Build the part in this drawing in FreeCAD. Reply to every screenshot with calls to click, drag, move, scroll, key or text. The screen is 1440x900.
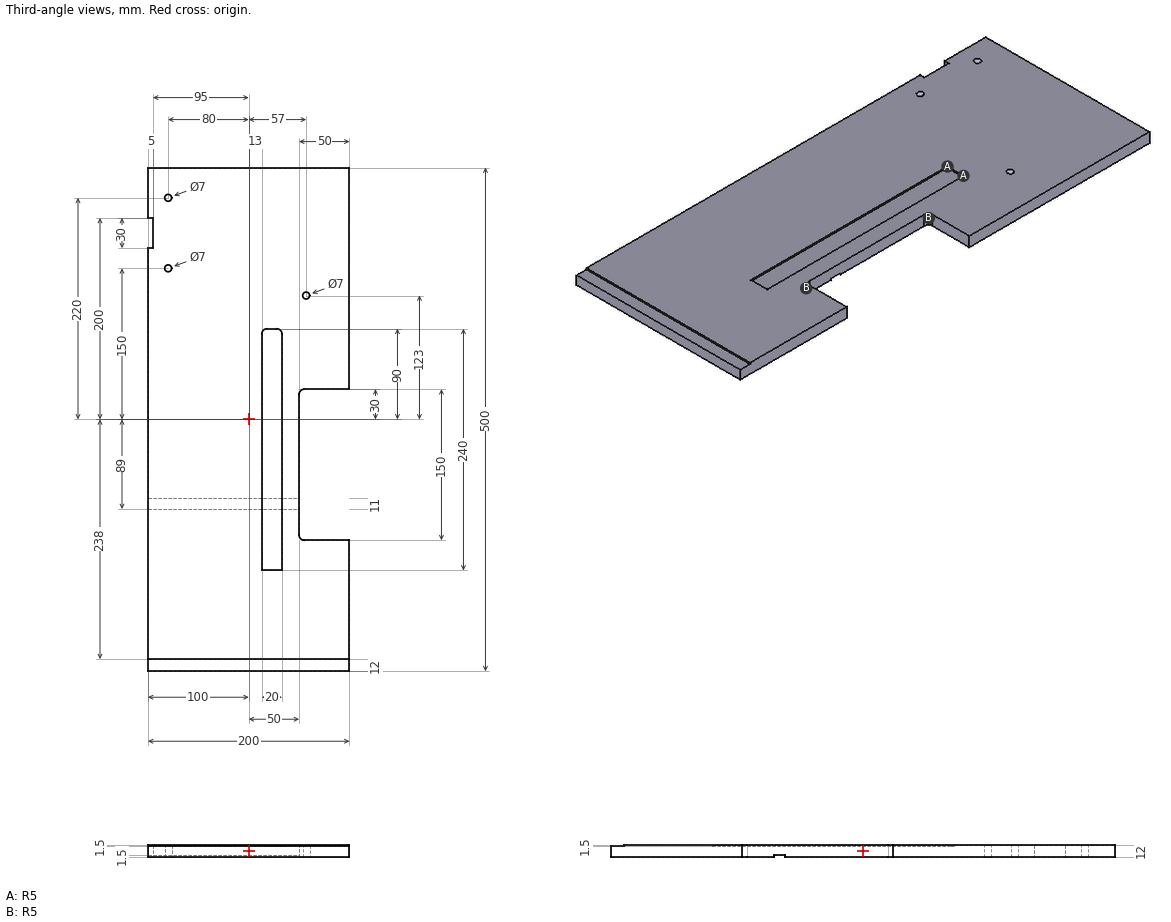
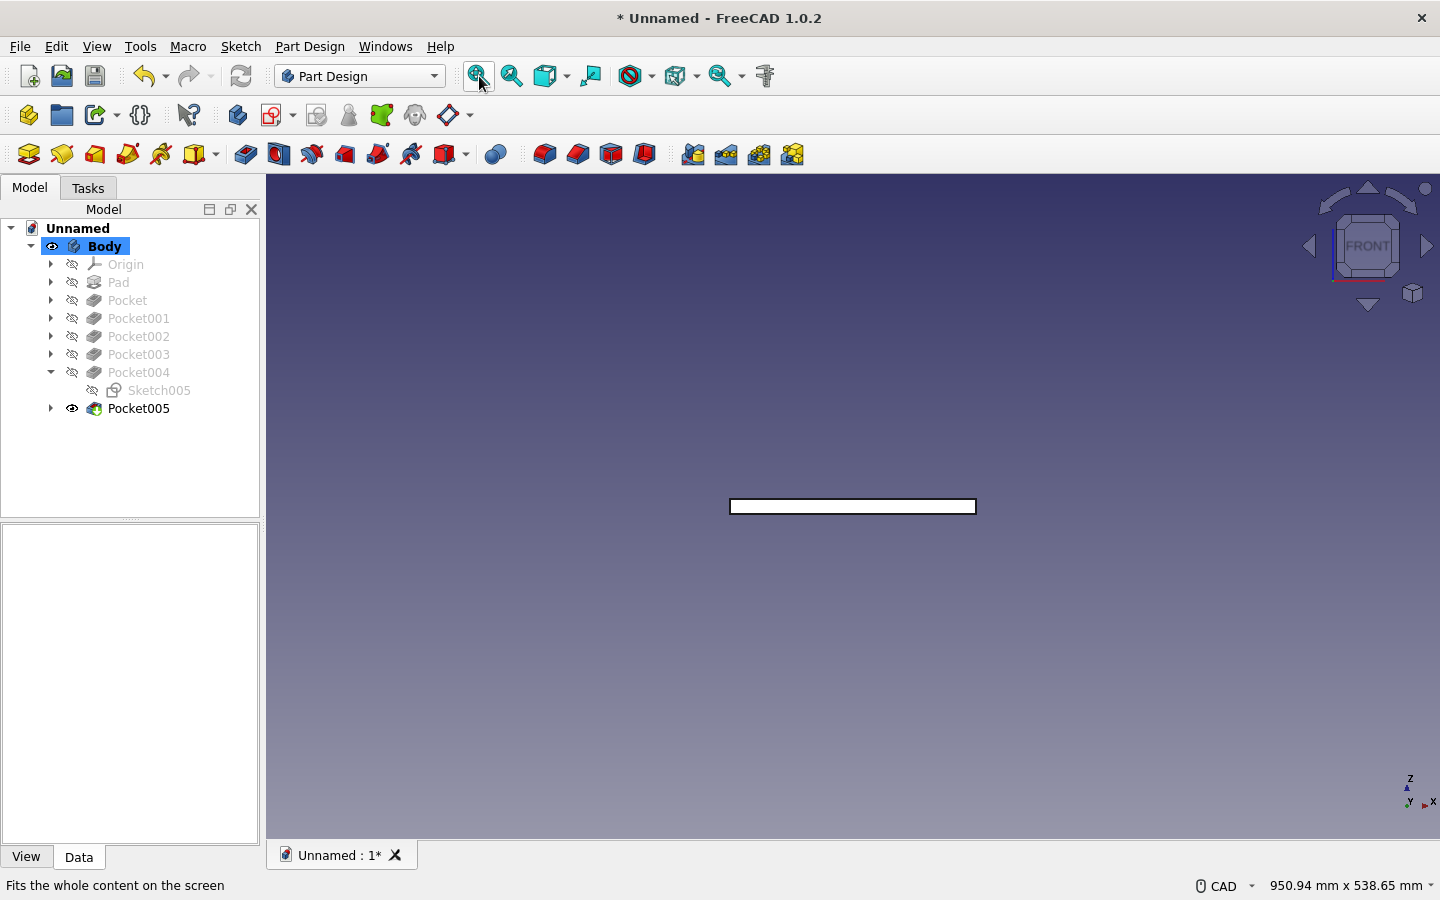
scroll(894, 499, up, 15)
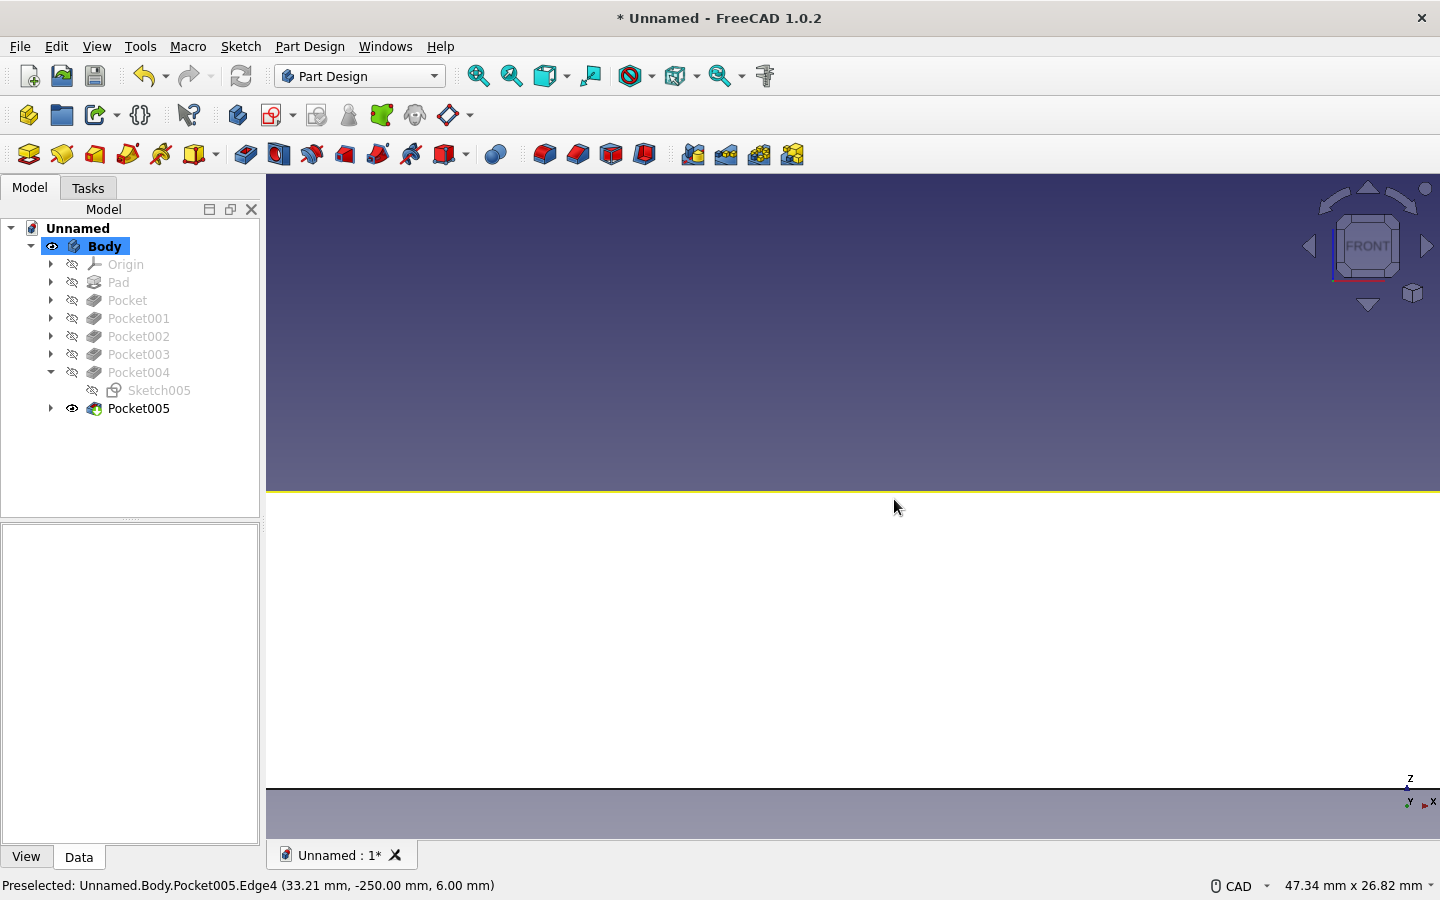
click(479, 76)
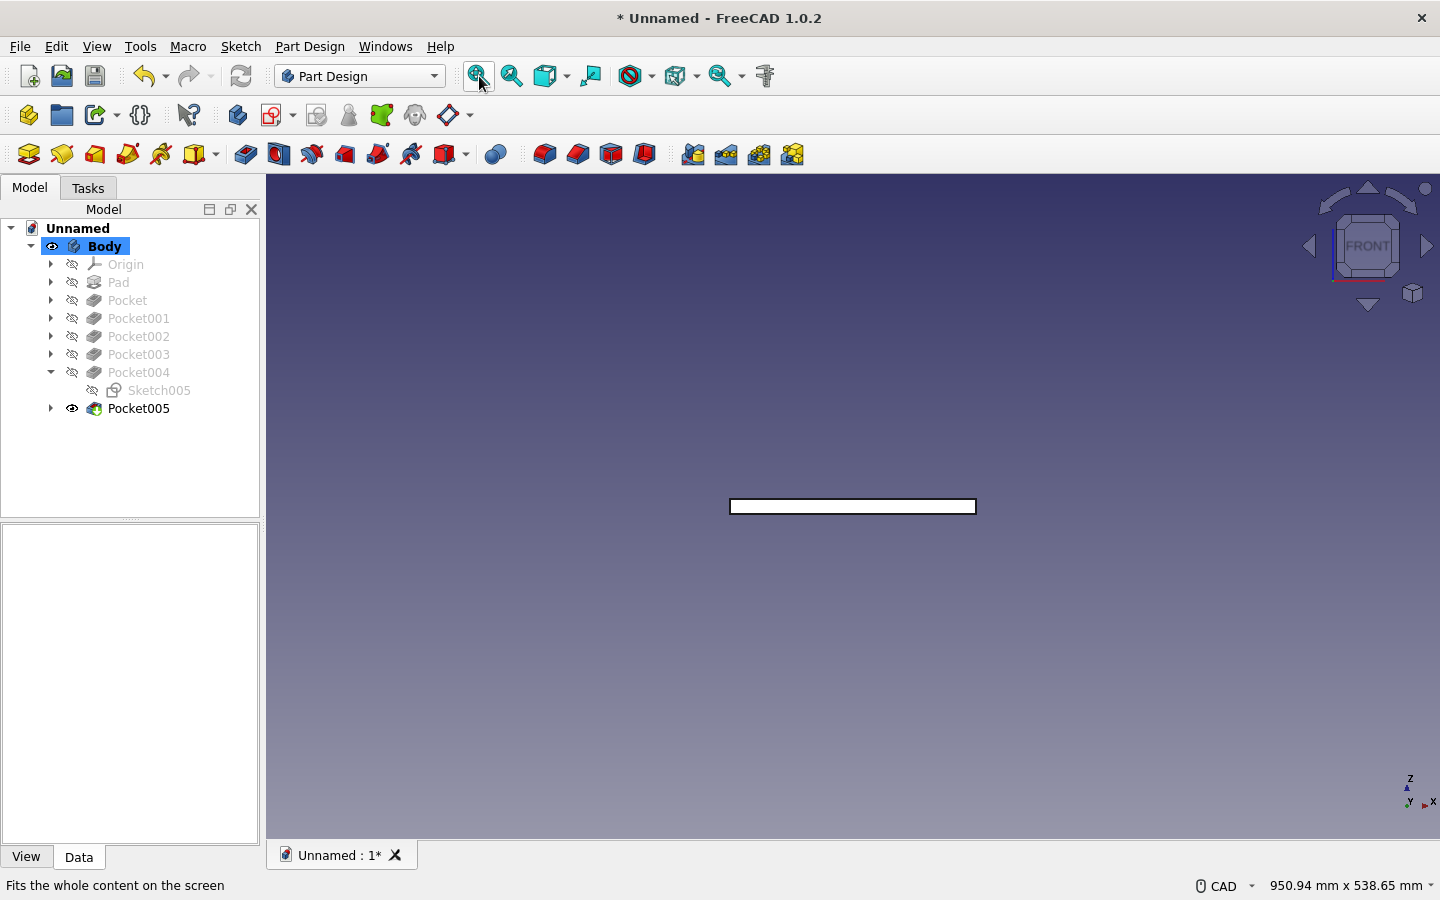
key(3)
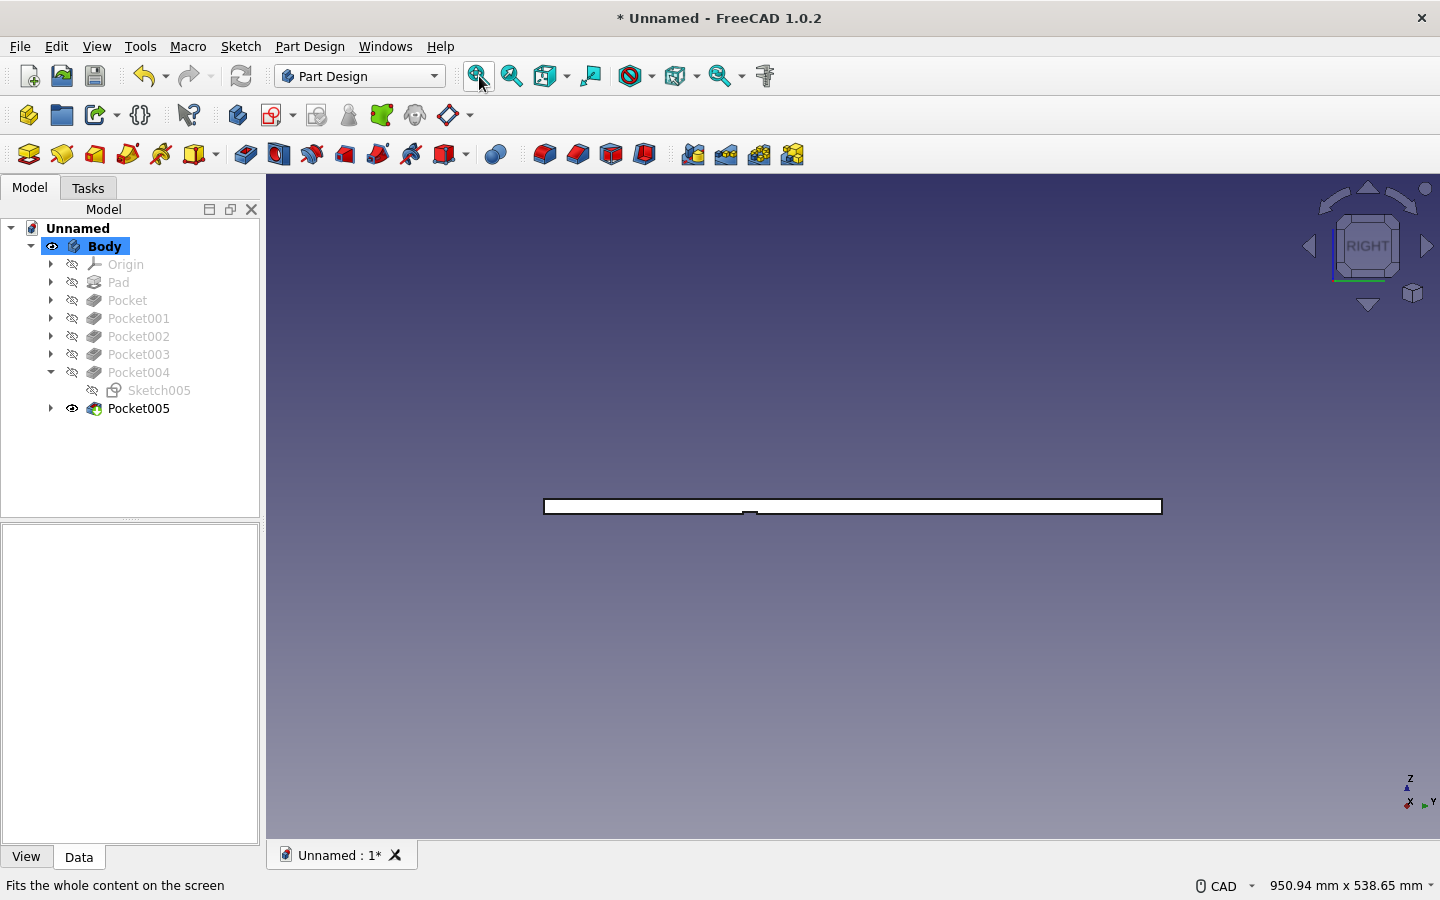
scroll(964, 499, up, 15)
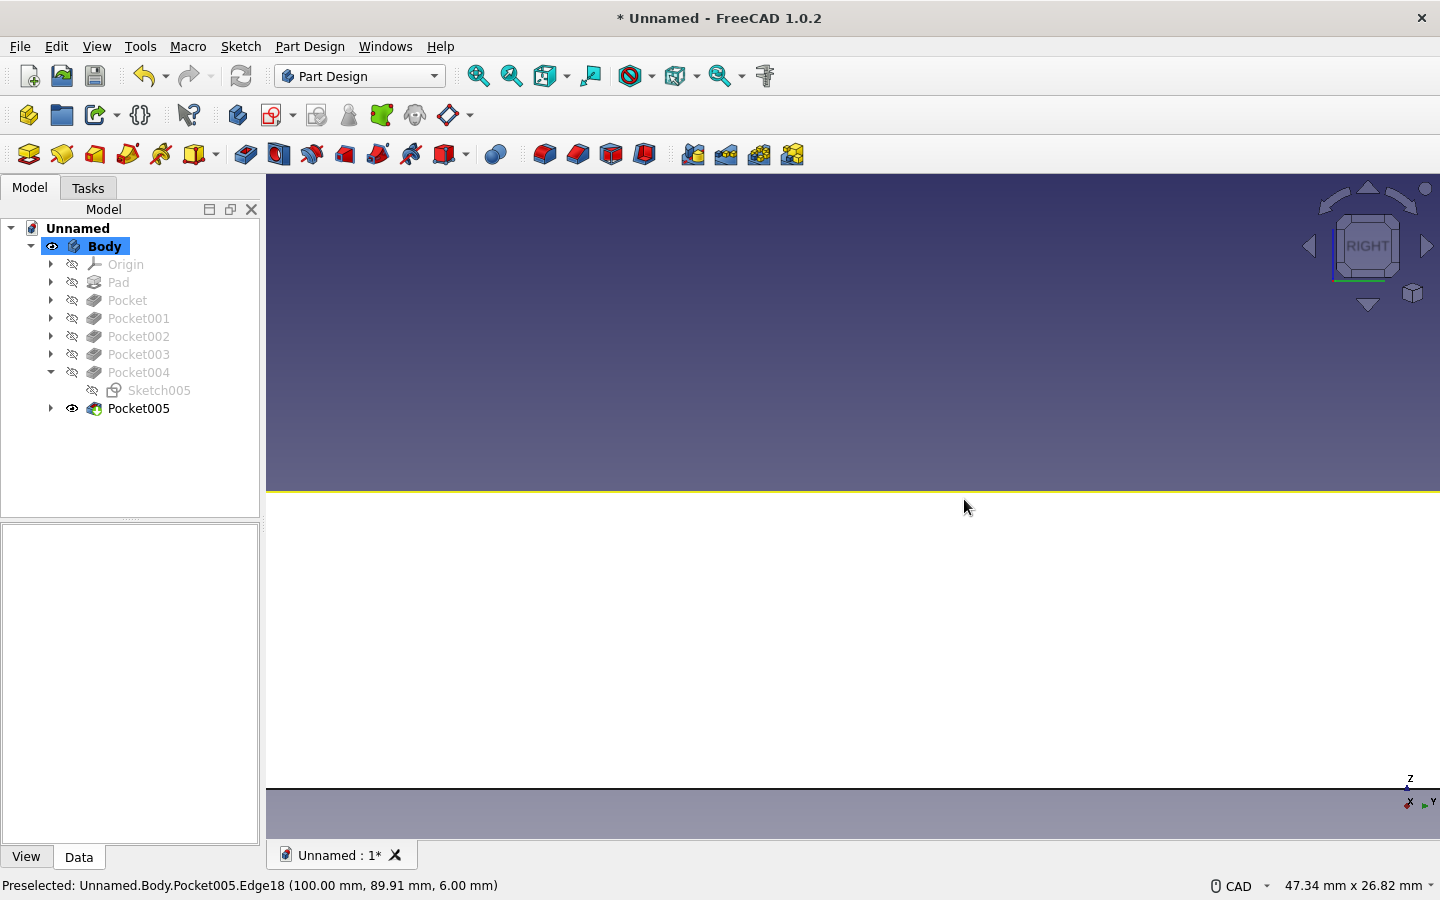
click(479, 76)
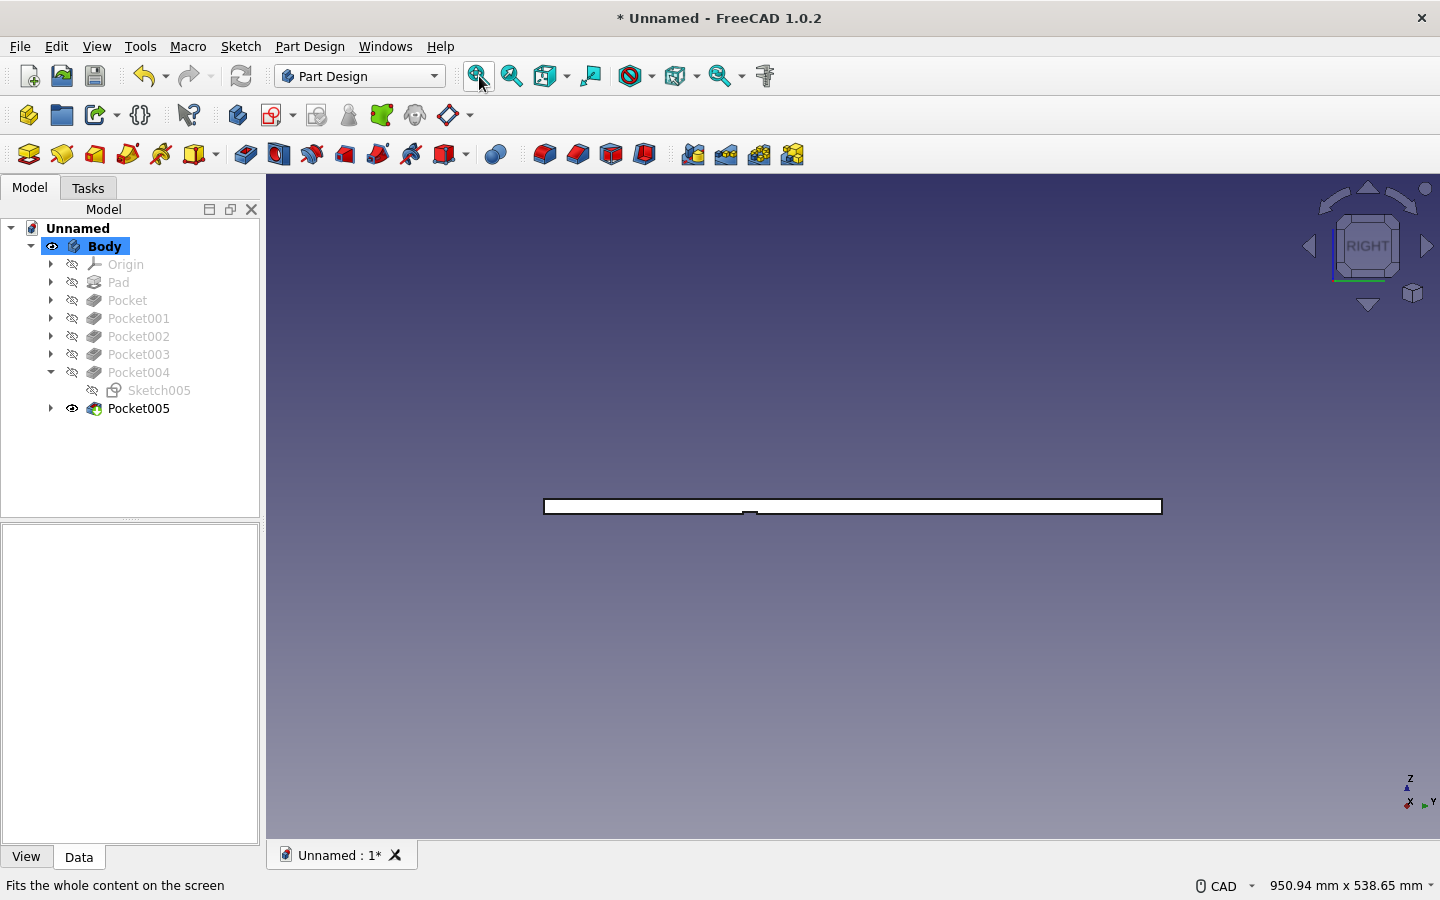
key(5)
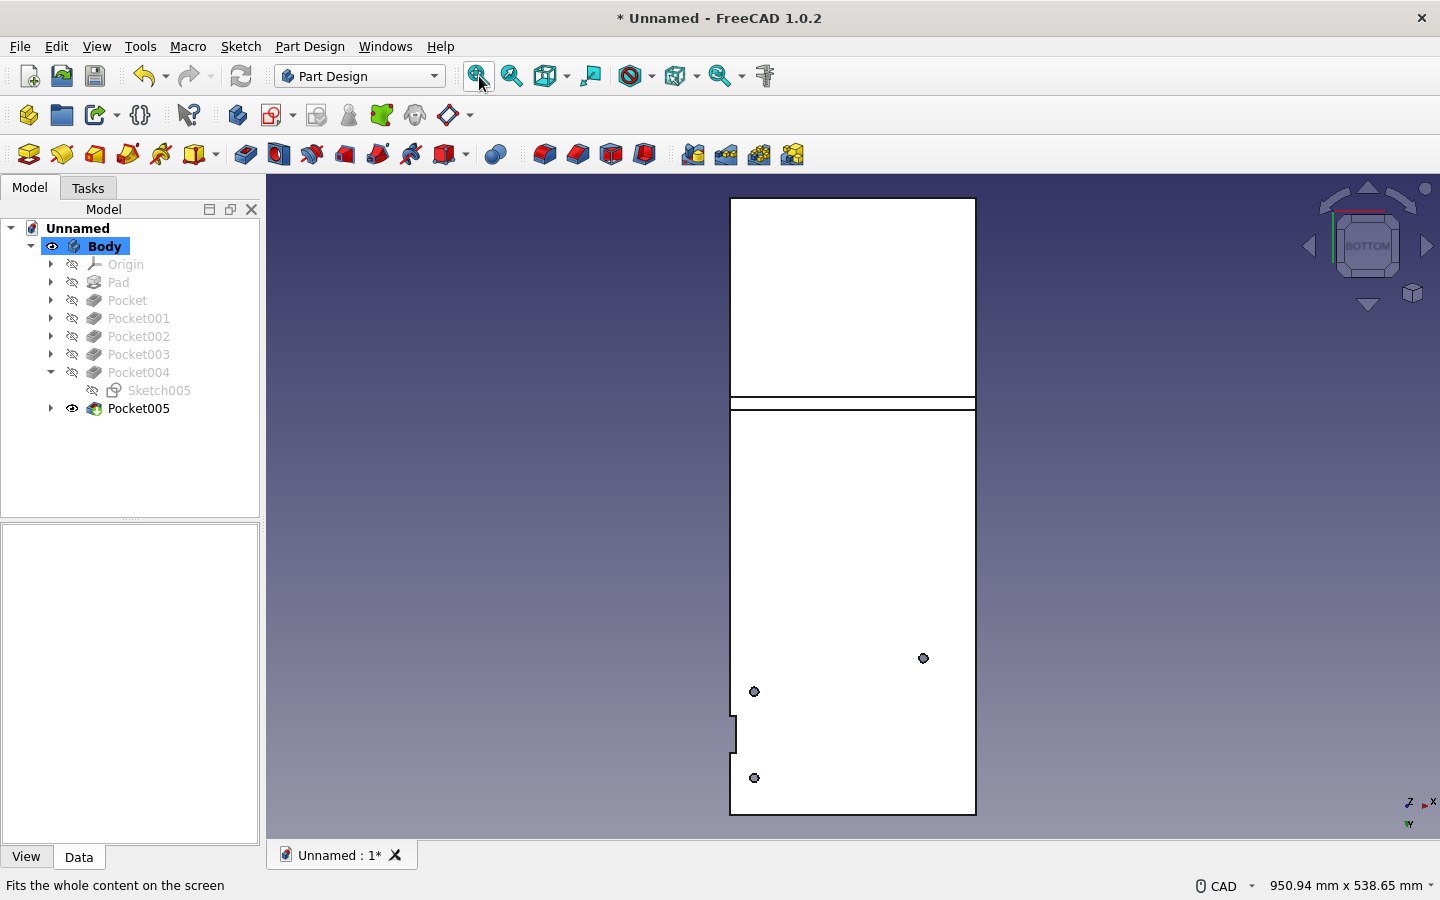
scroll(894, 617, up, 15)